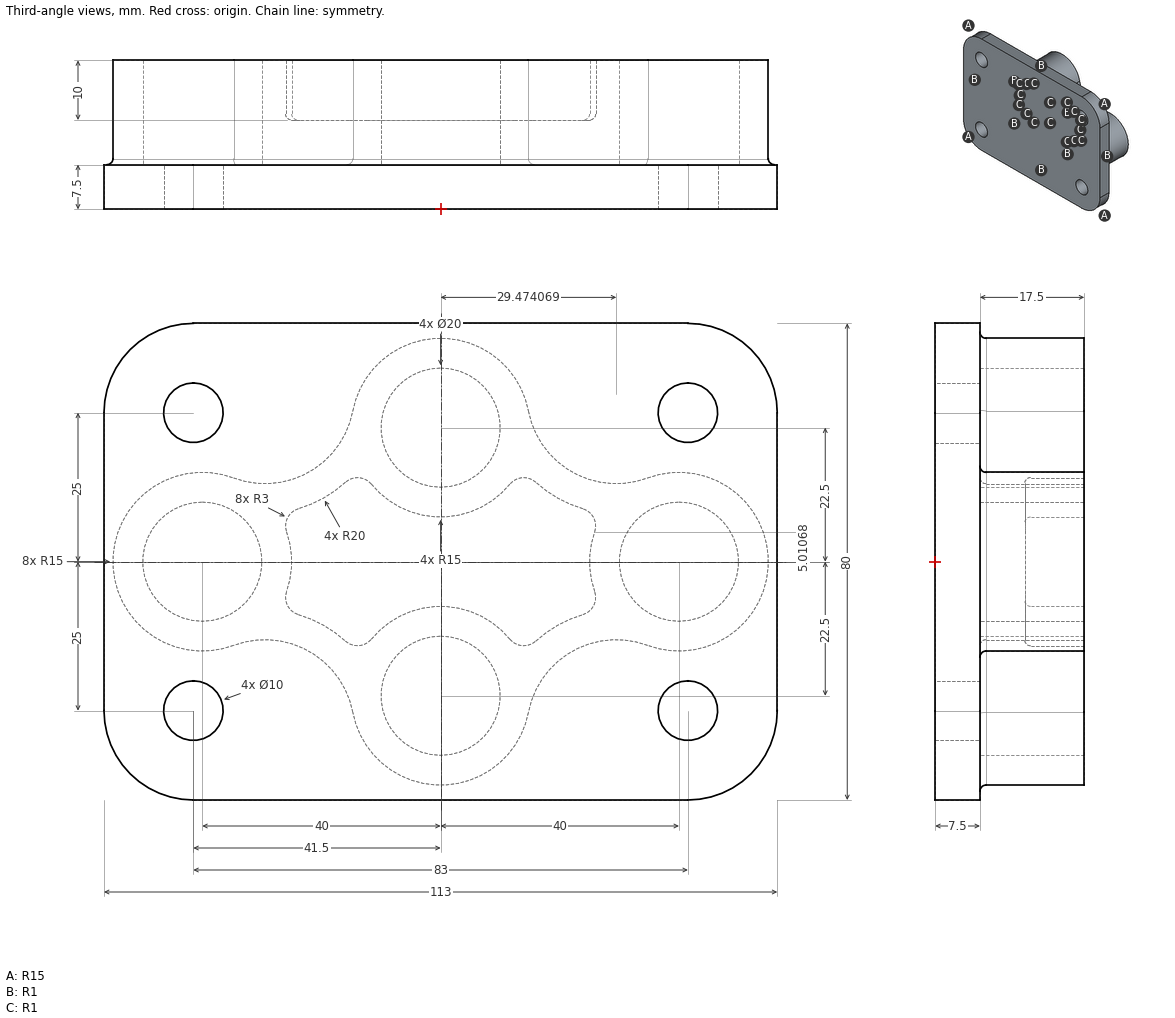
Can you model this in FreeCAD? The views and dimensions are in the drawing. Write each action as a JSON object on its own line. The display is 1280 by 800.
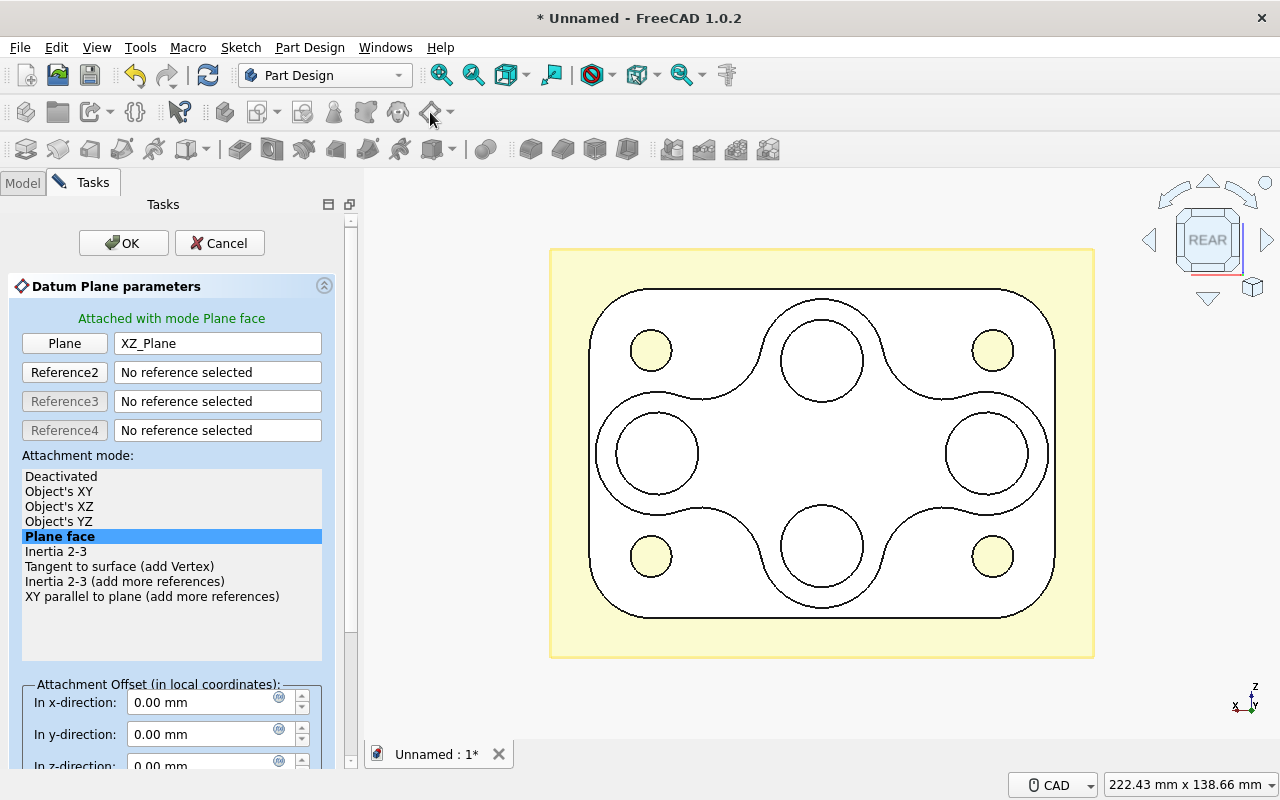
{"action": "scroll", "coordinate": [351, 491], "scroll_direction": "down", "scroll_amount": 2}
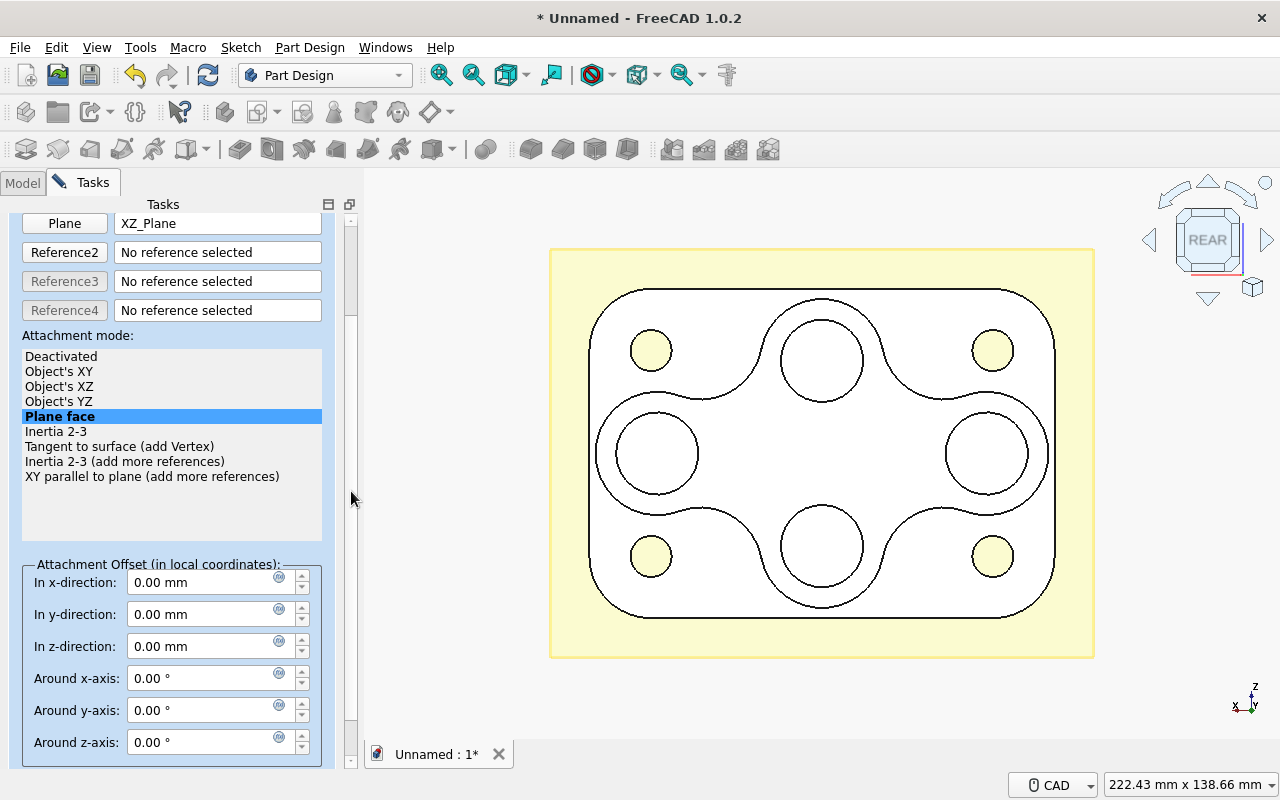
{"action": "triple_click", "coordinate": [210, 646]}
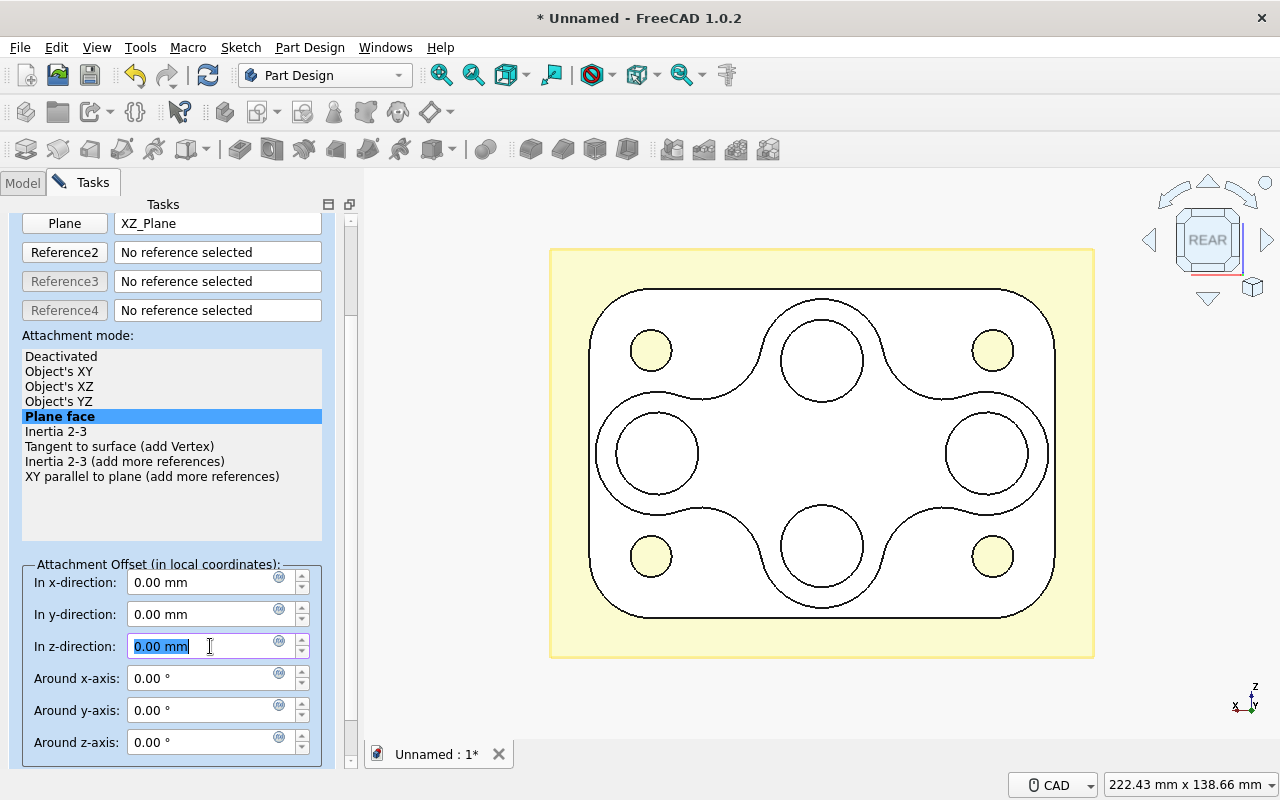
{"action": "type", "text": "-15"}
{"action": "key", "text": "Tab"}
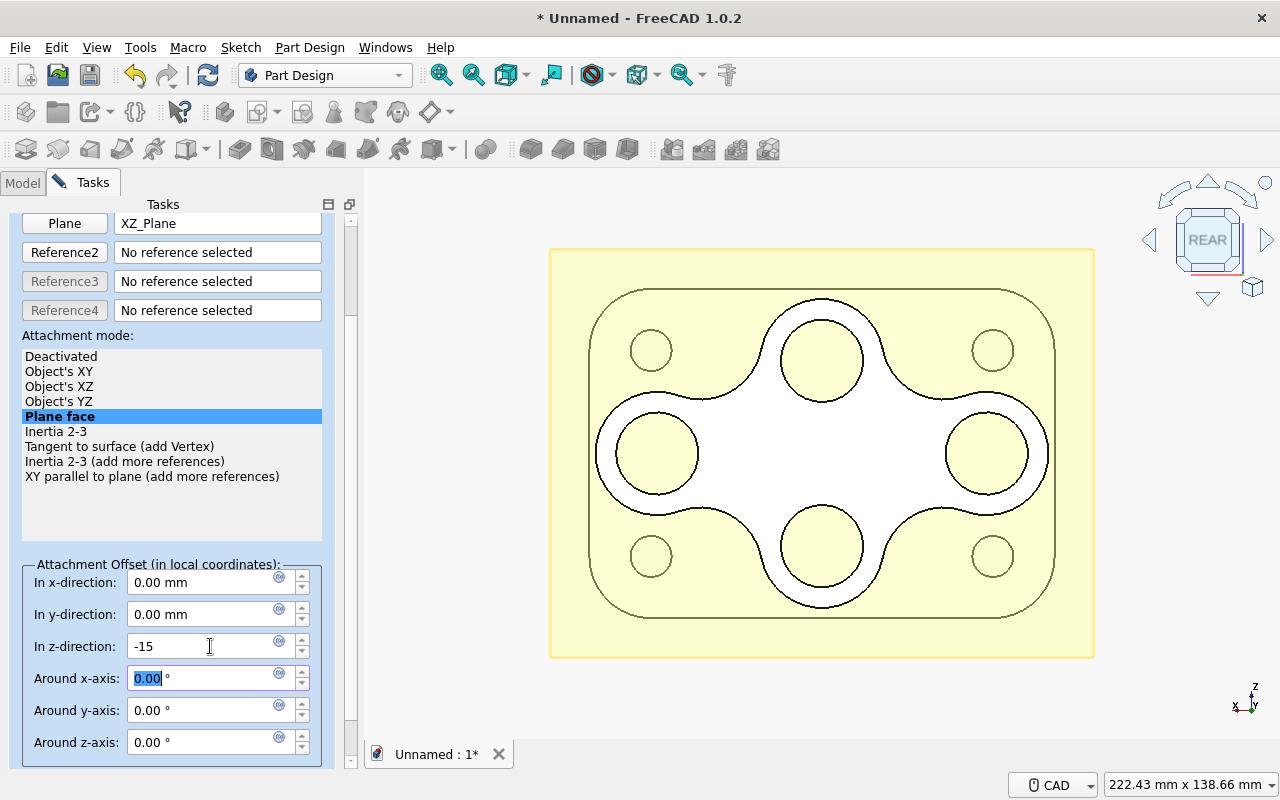
{"action": "scroll", "coordinate": [351, 491], "scroll_direction": "up", "scroll_amount": 3}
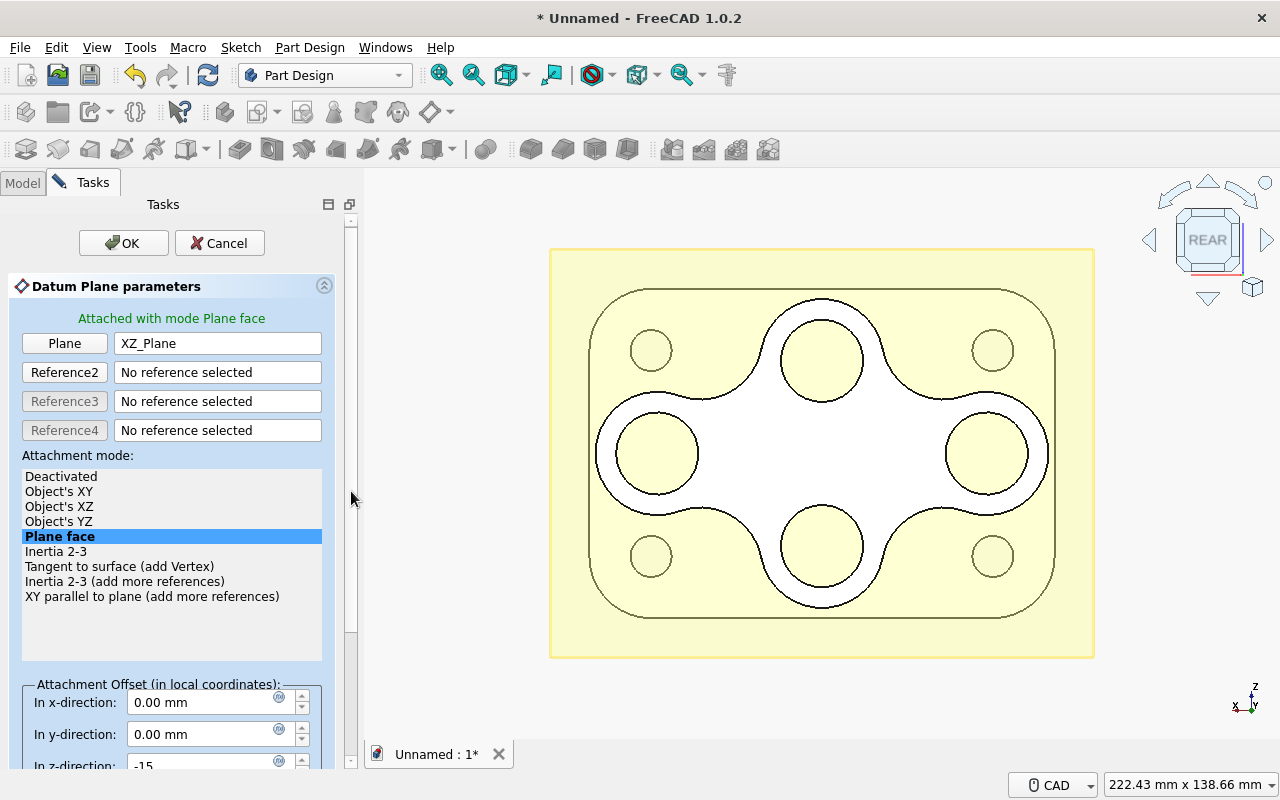
{"action": "left_click", "coordinate": [124, 243]}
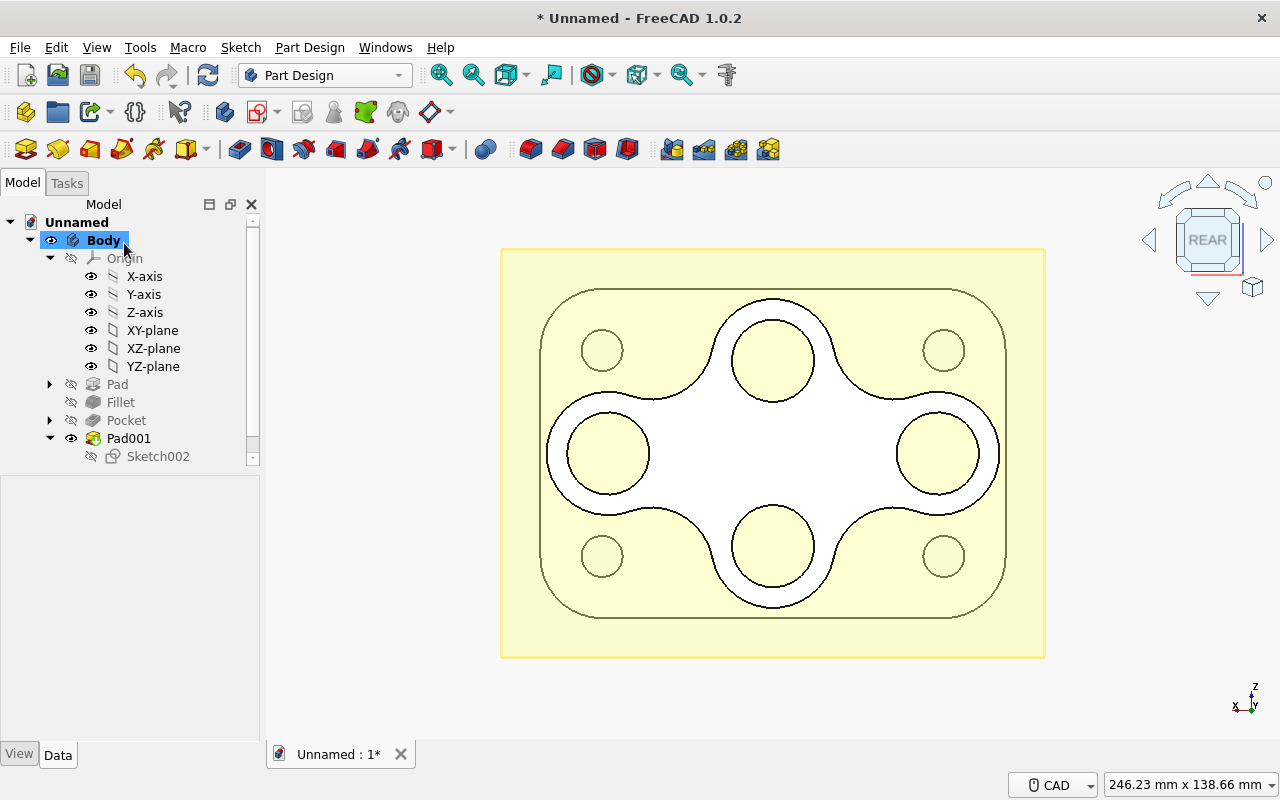
{"action": "scroll", "coordinate": [100, 344], "scroll_direction": "down", "scroll_amount": 3}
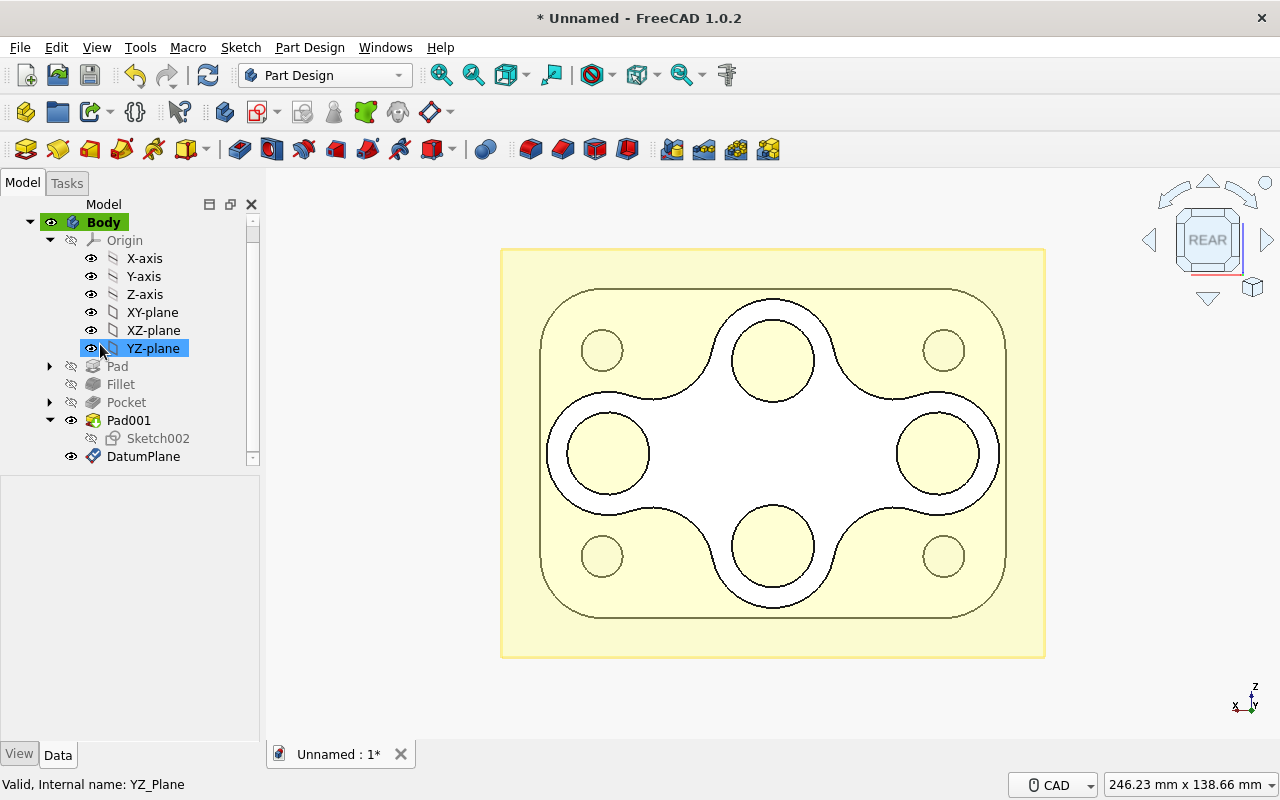
{"action": "left_click", "coordinate": [116, 456]}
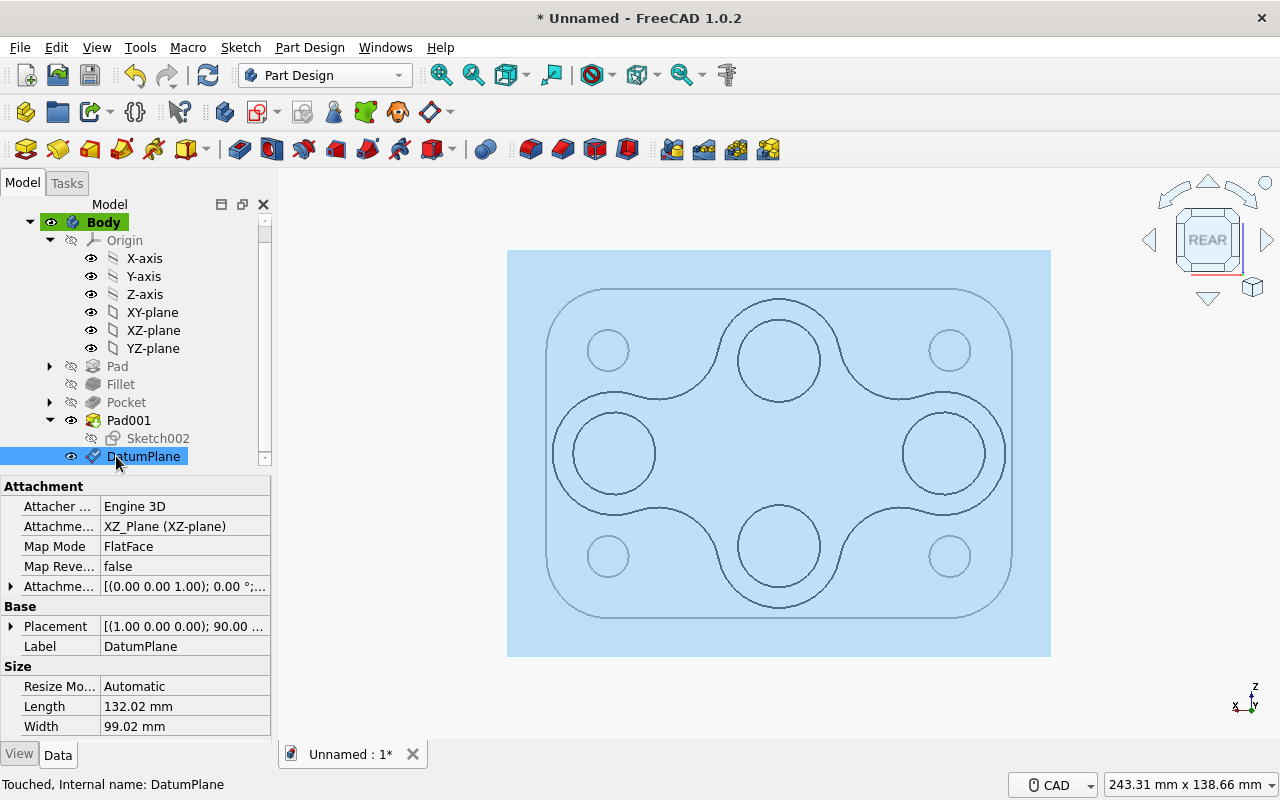
{"action": "left_click", "coordinate": [258, 112]}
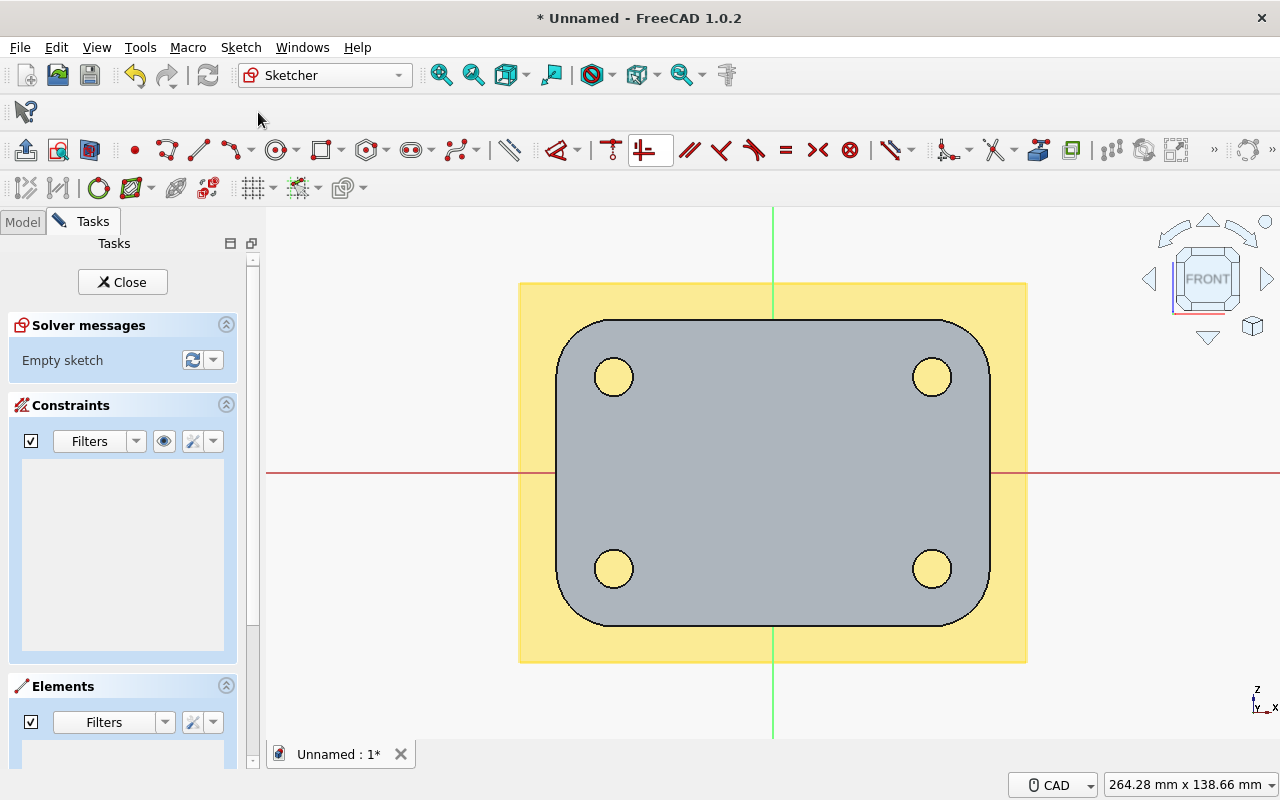
{"action": "key", "text": "q s"}